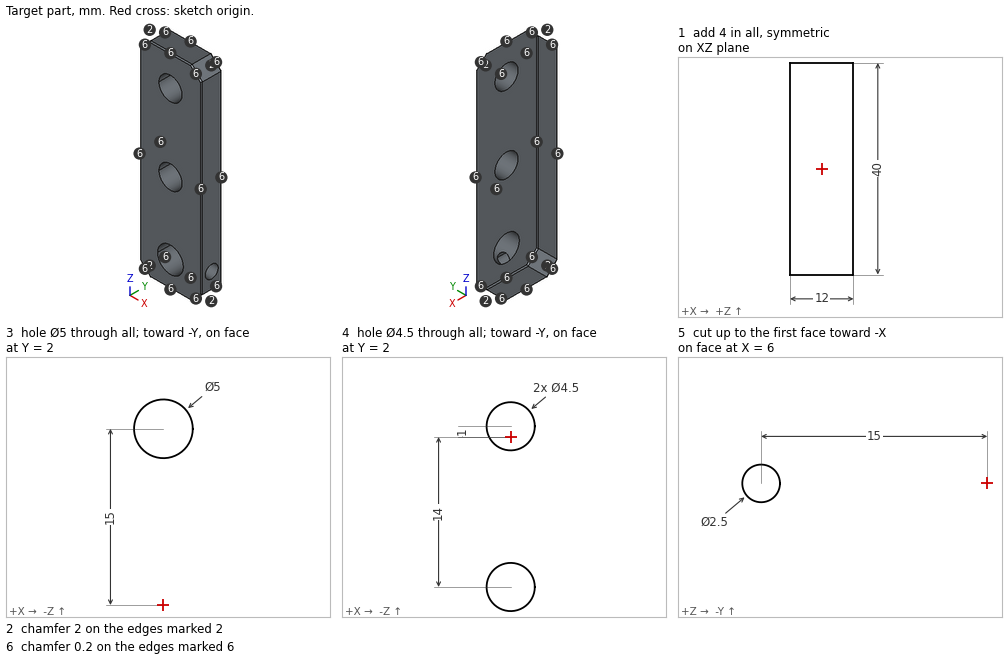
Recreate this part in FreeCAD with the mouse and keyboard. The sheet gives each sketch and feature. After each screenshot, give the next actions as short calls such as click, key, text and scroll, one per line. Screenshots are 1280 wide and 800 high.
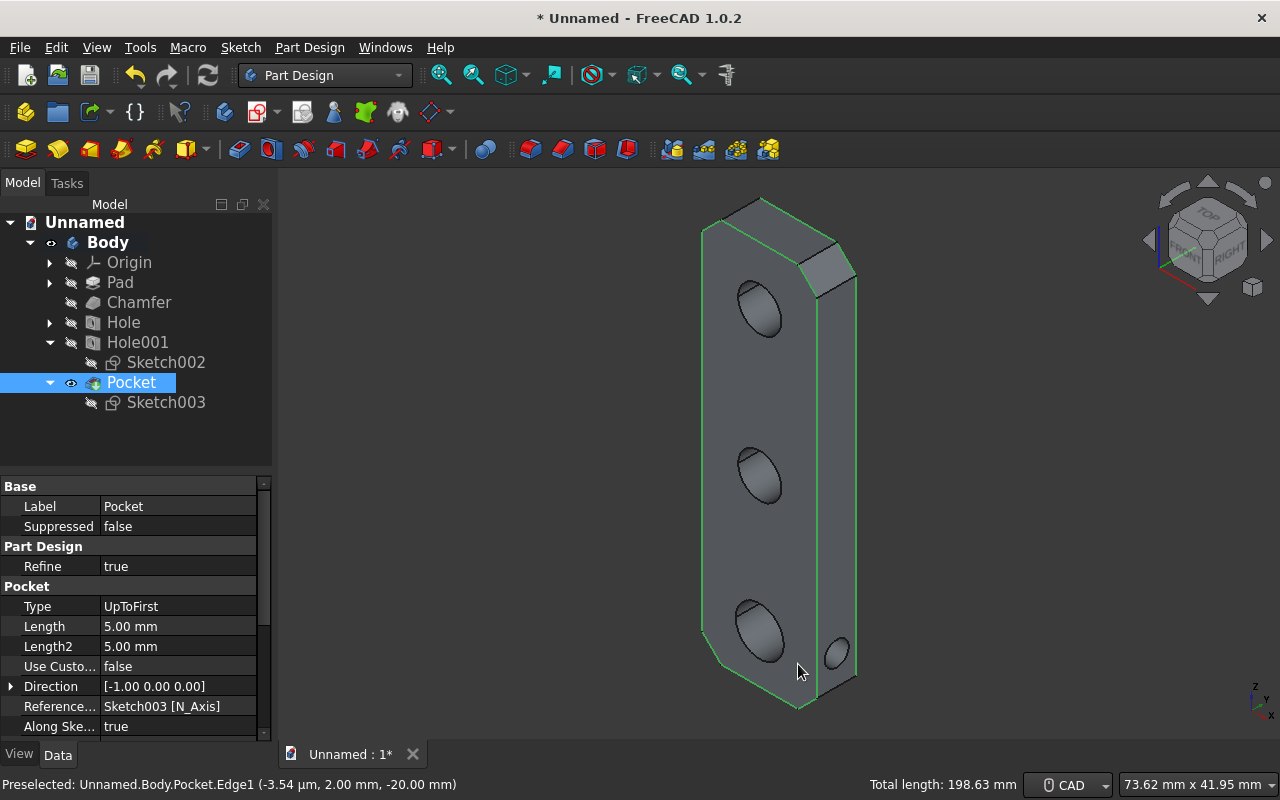
click(564, 150)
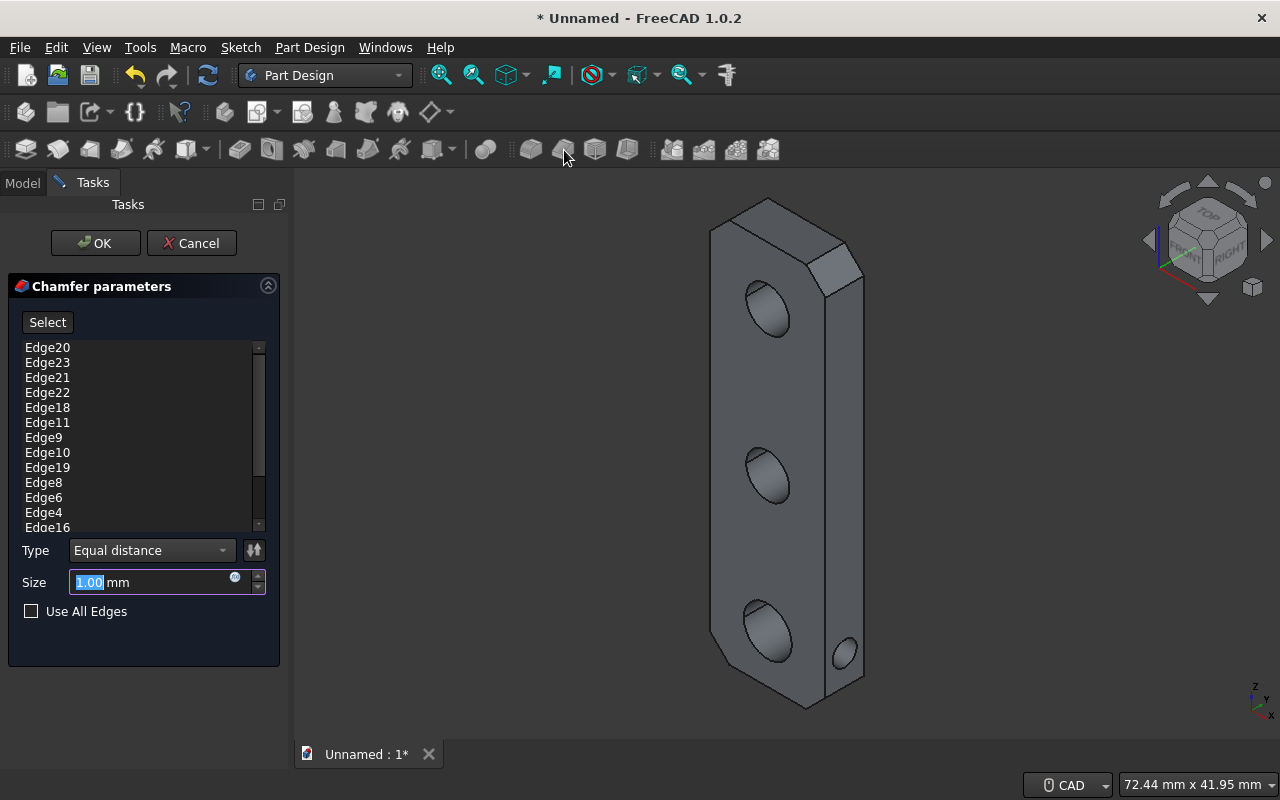
text(0.2)
key(Tab)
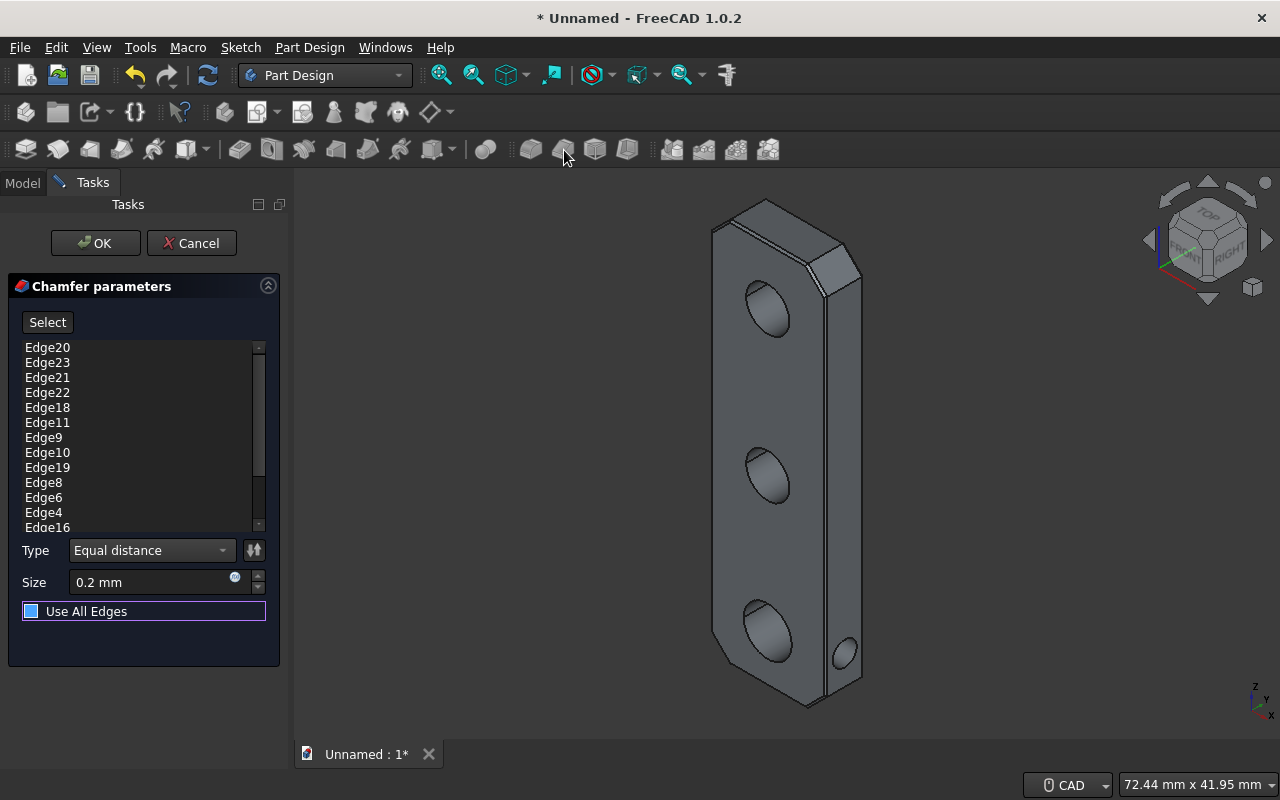
click(96, 243)